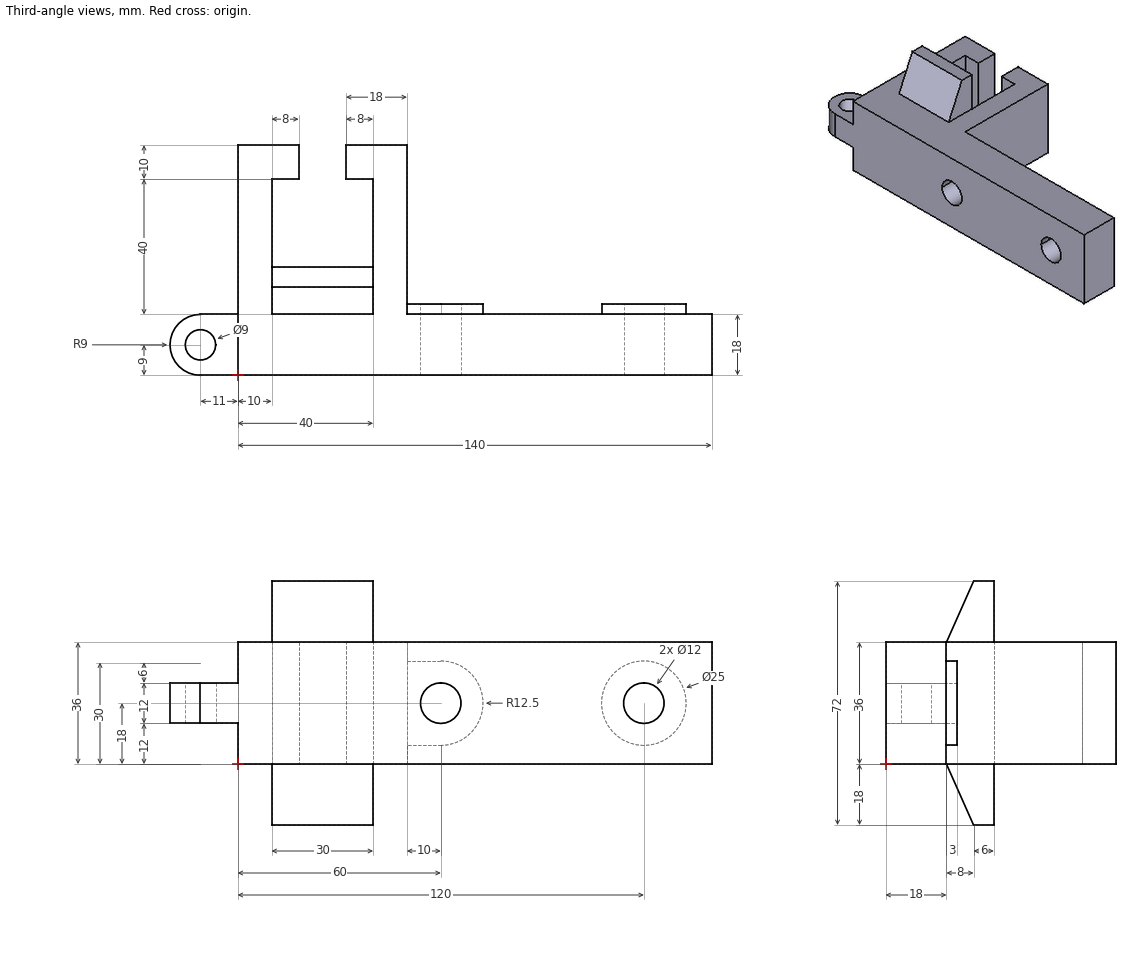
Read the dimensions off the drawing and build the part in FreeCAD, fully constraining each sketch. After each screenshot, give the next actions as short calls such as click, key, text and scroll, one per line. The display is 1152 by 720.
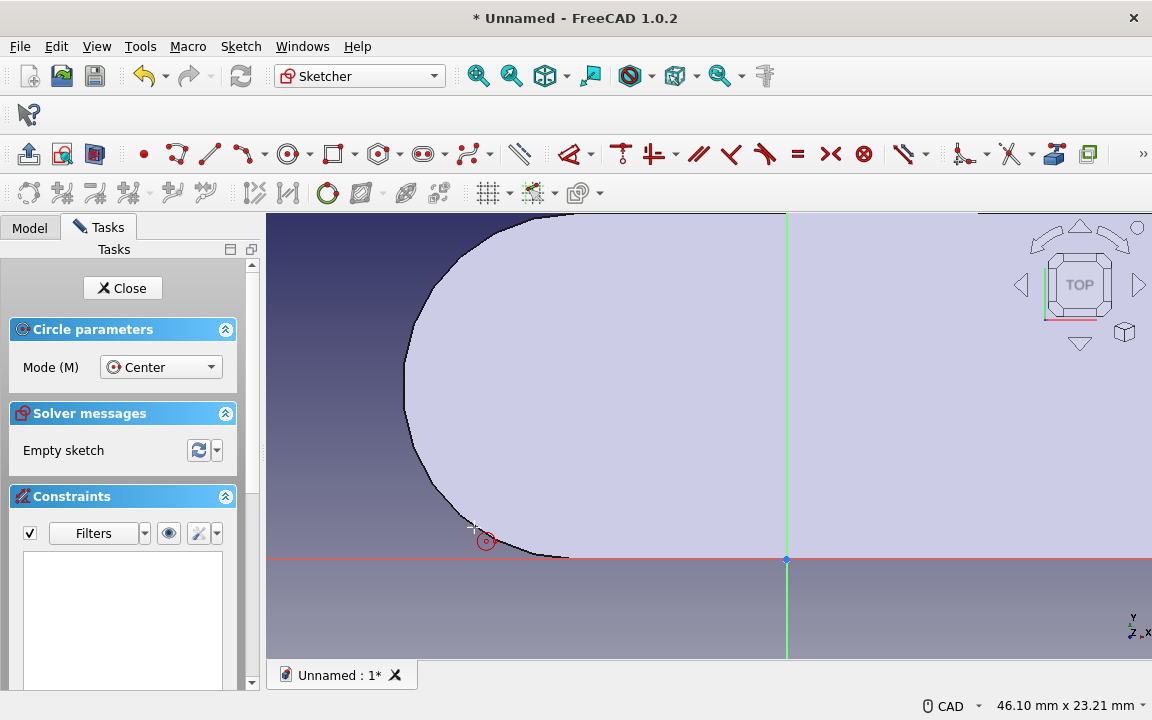
click(575, 386)
click(636, 325)
key(Escape)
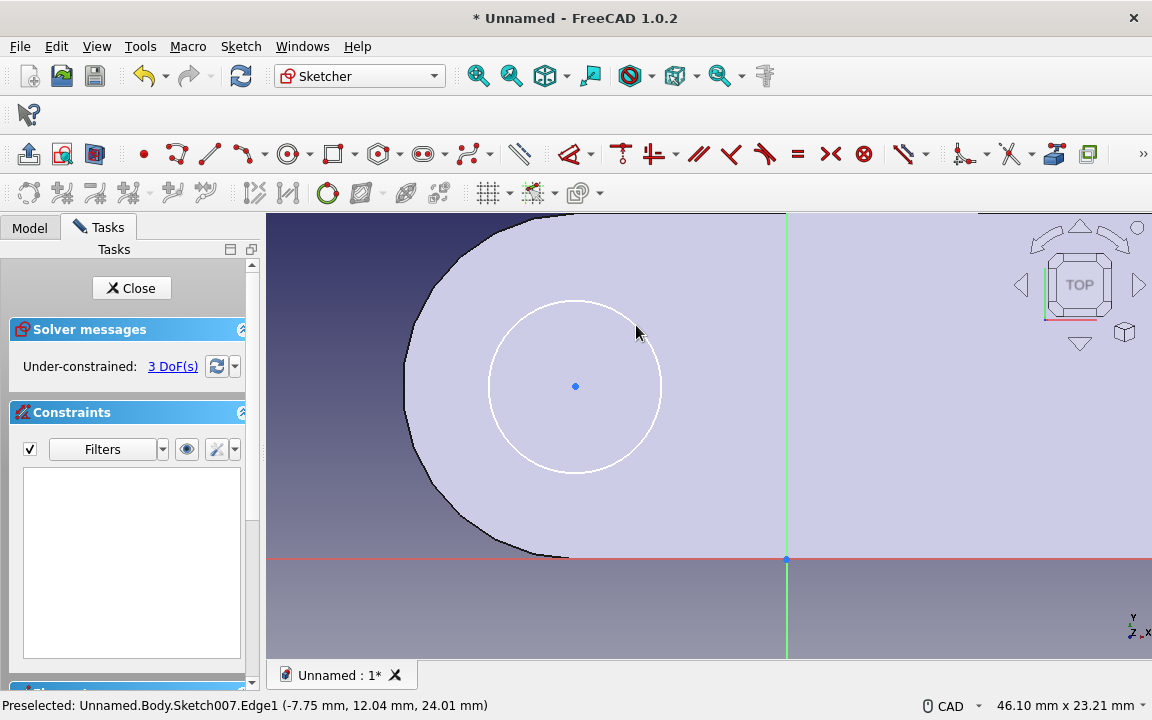
click(568, 154)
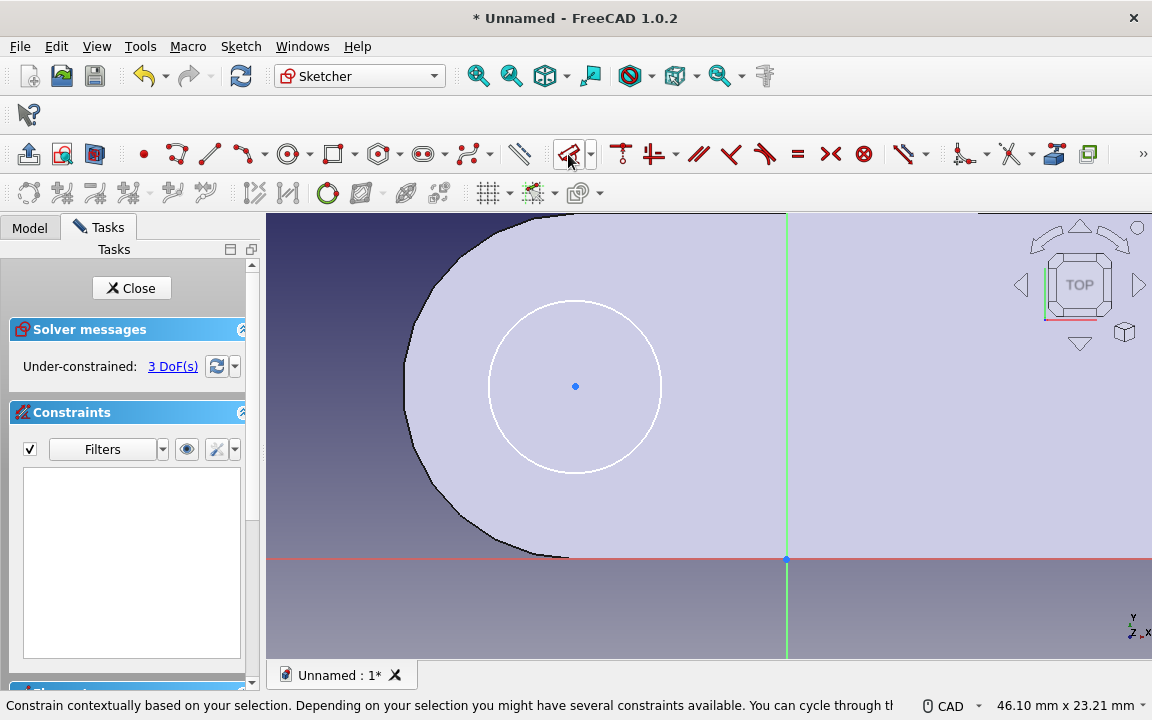
click(636, 326)
click(659, 303)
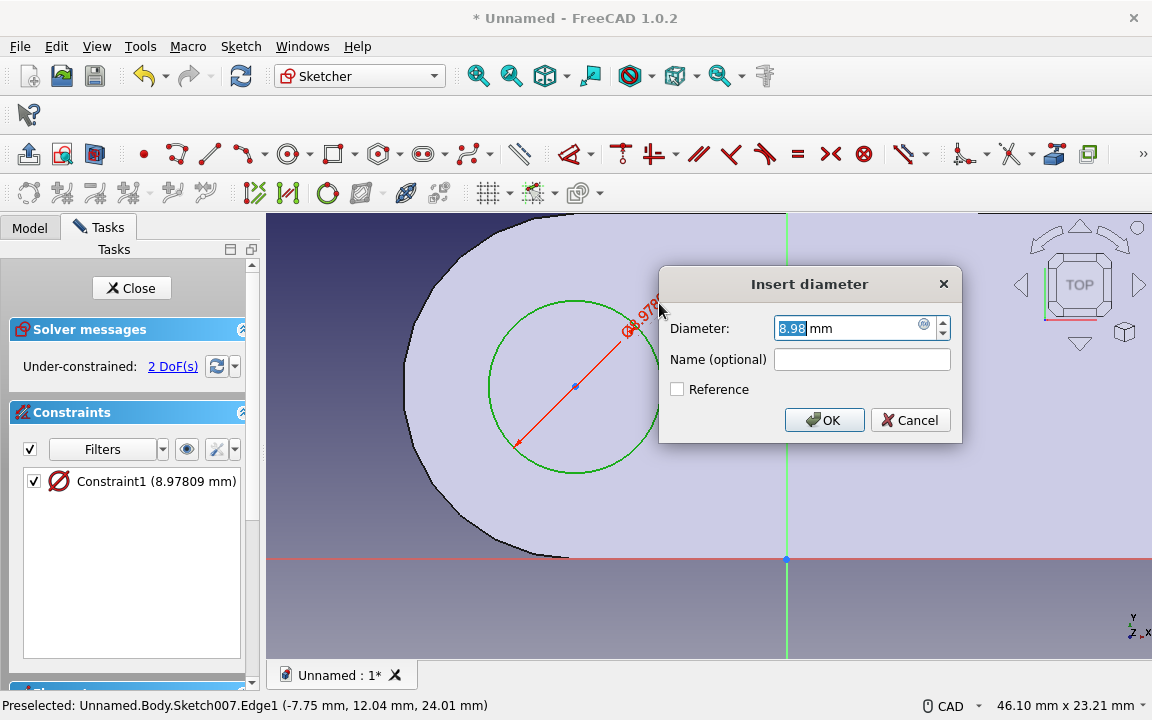
text(9)
key(Return)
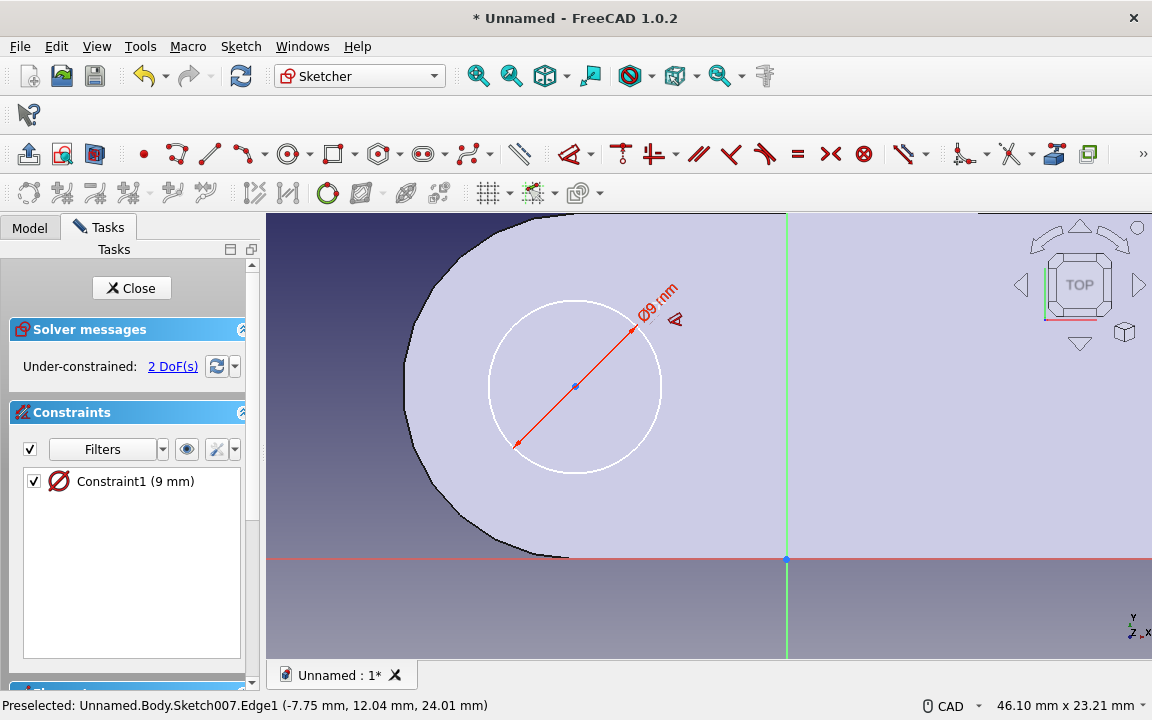
click(575, 387)
click(821, 473)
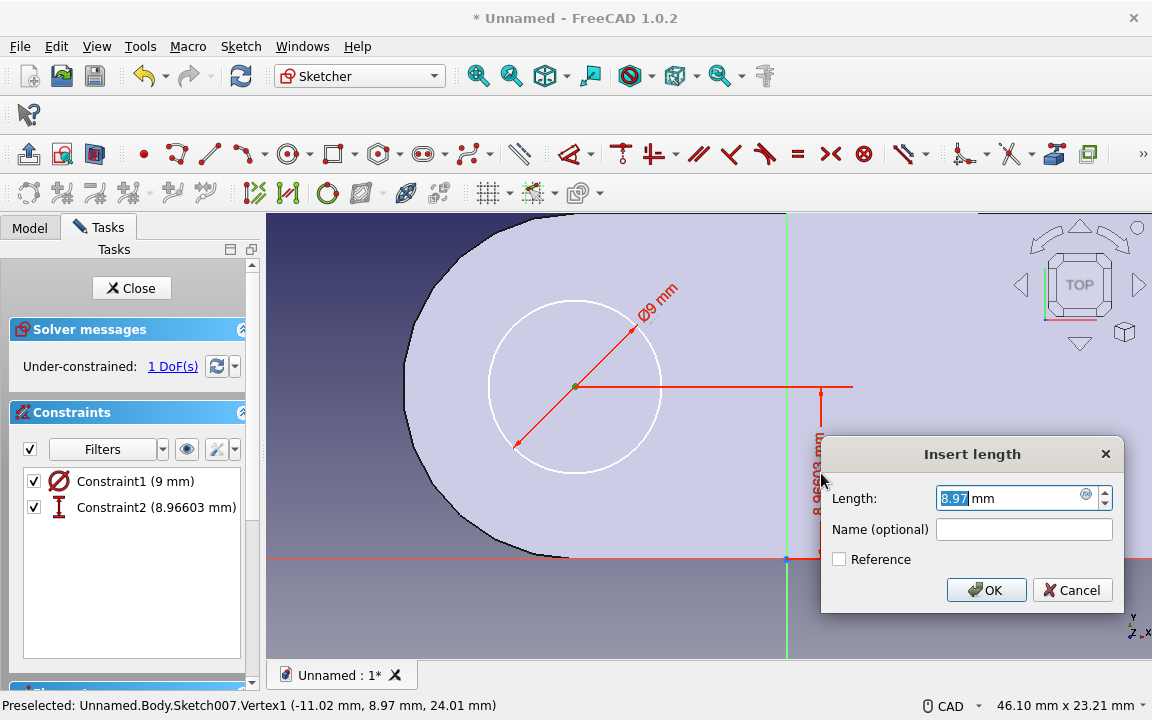
text(9)
key(Return)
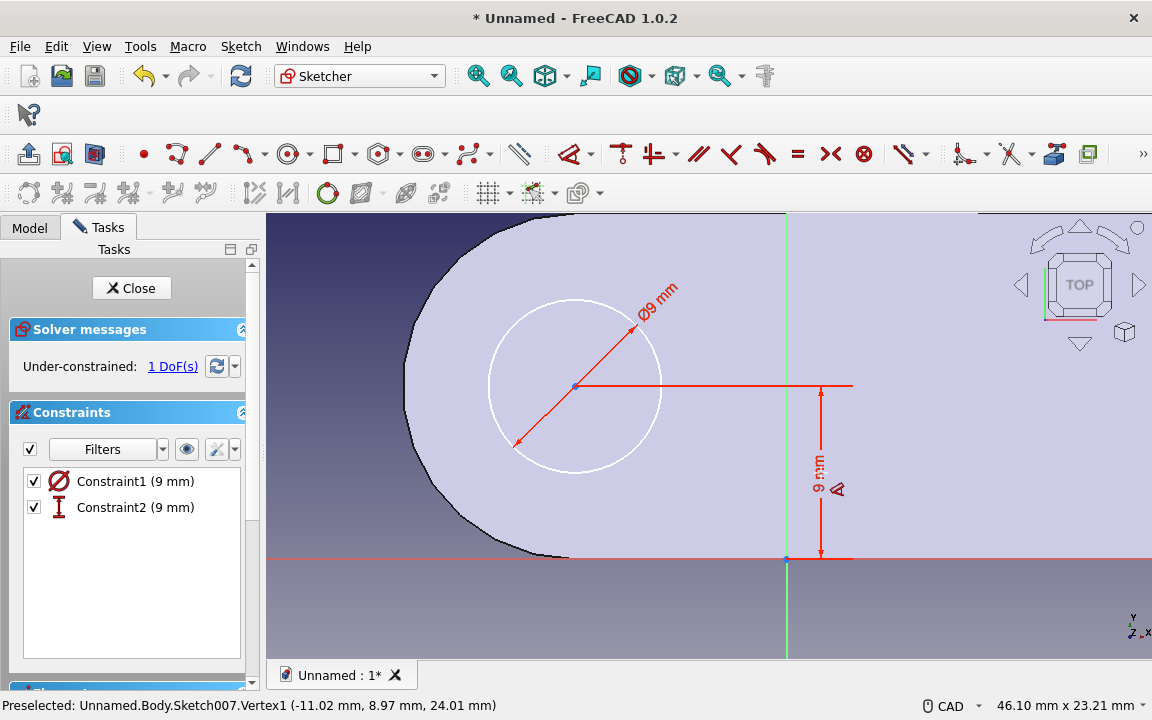
click(575, 386)
click(681, 593)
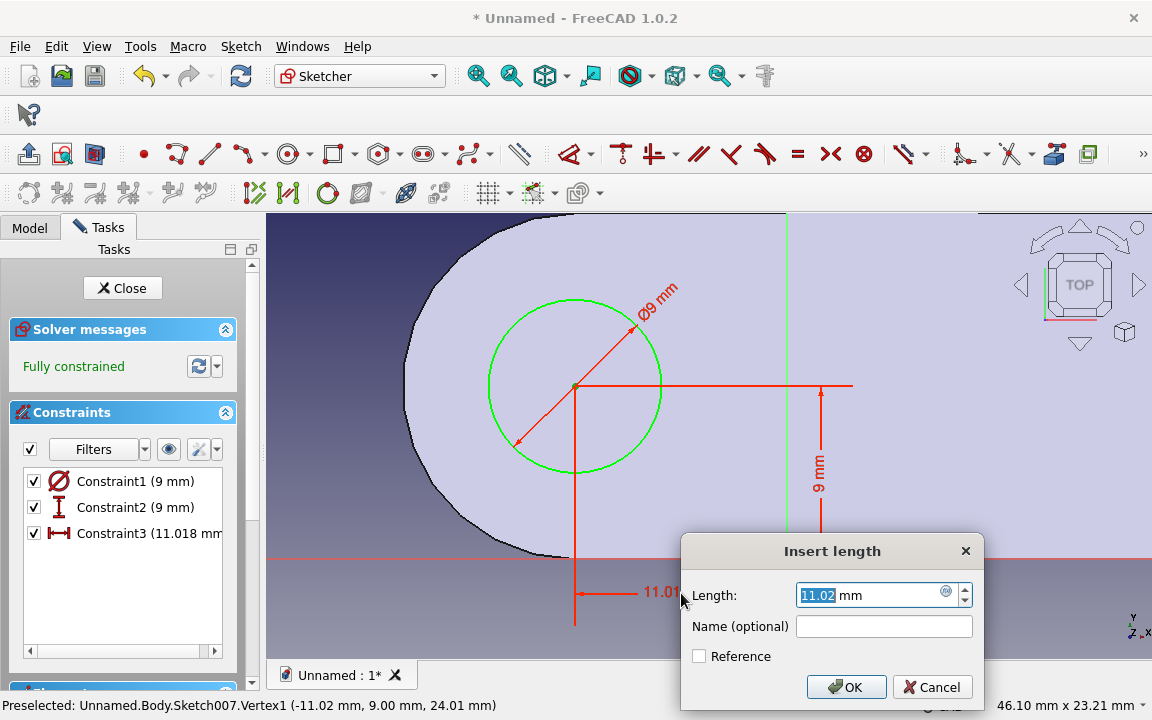
text(11)
key(Return)
key(Escape)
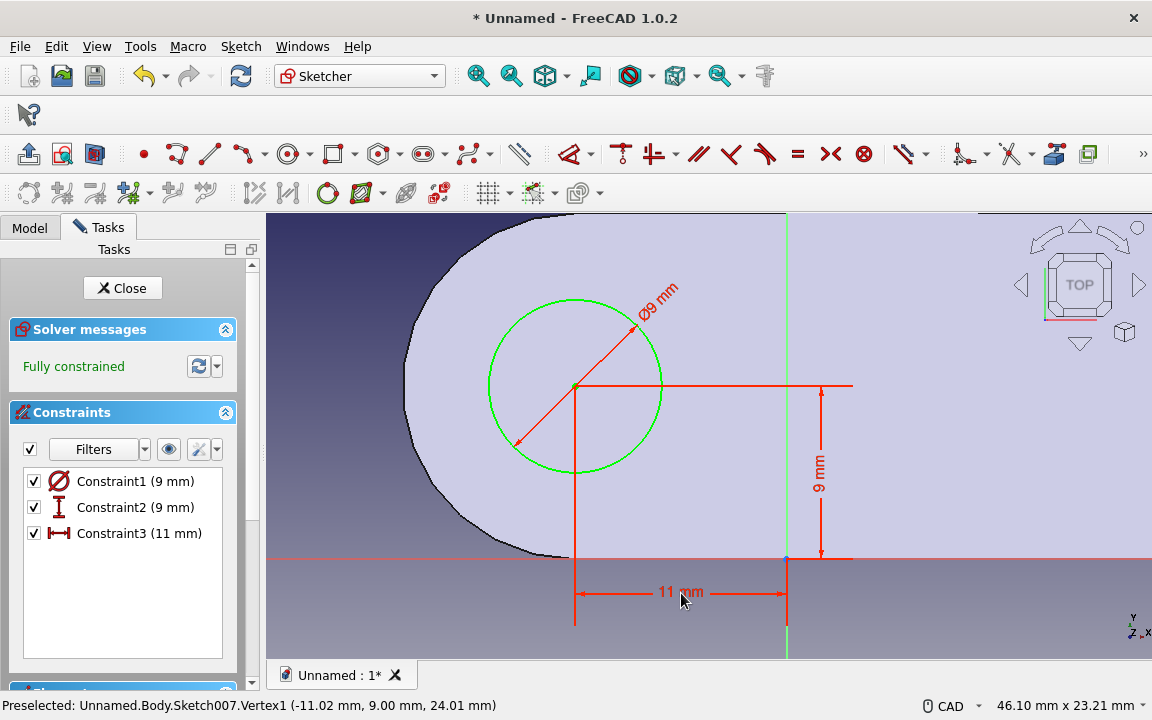
click(123, 288)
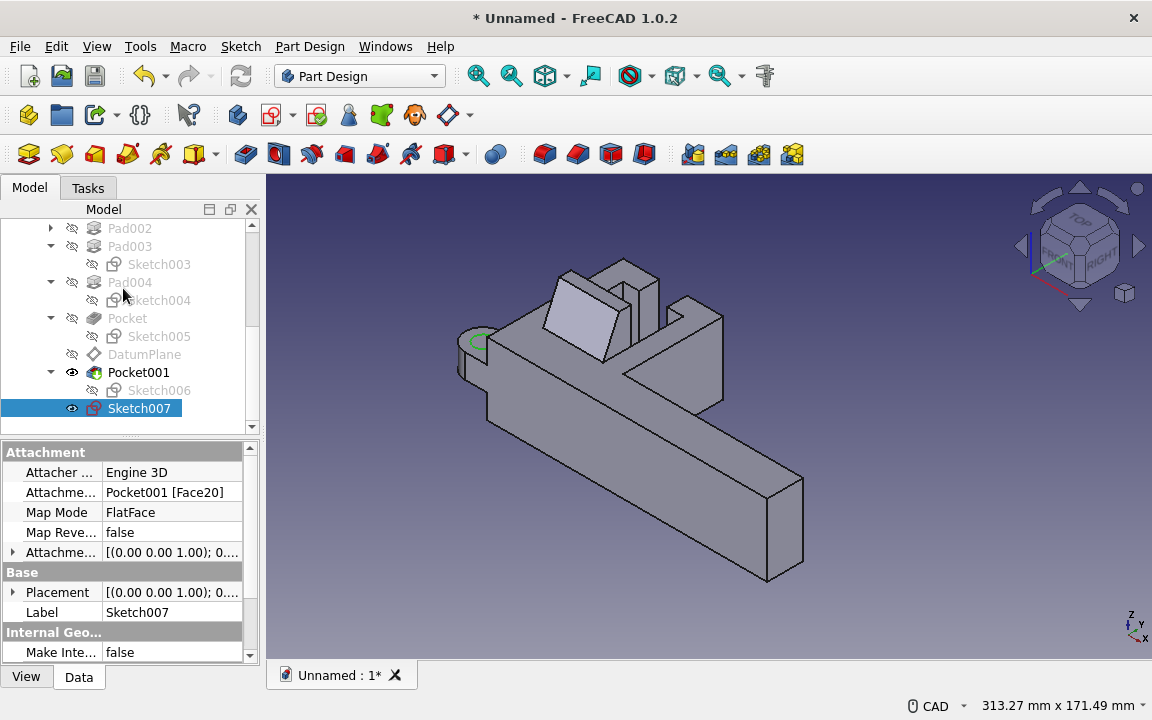
click(246, 154)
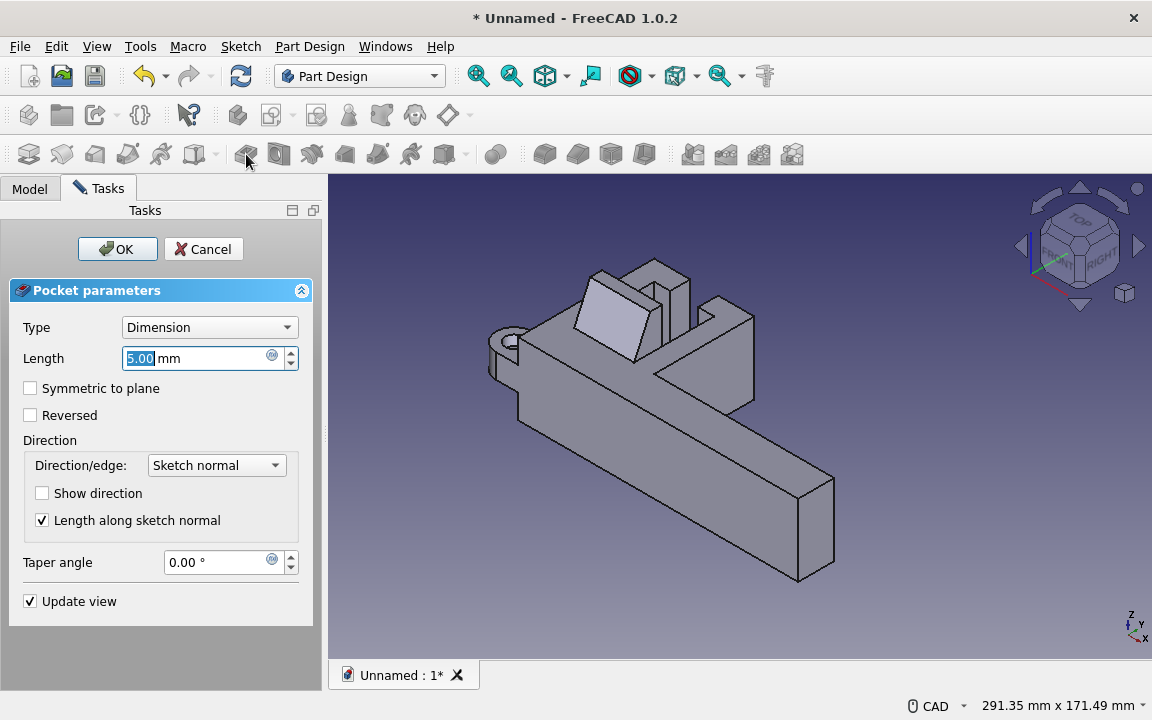
text(12)
key(Tab)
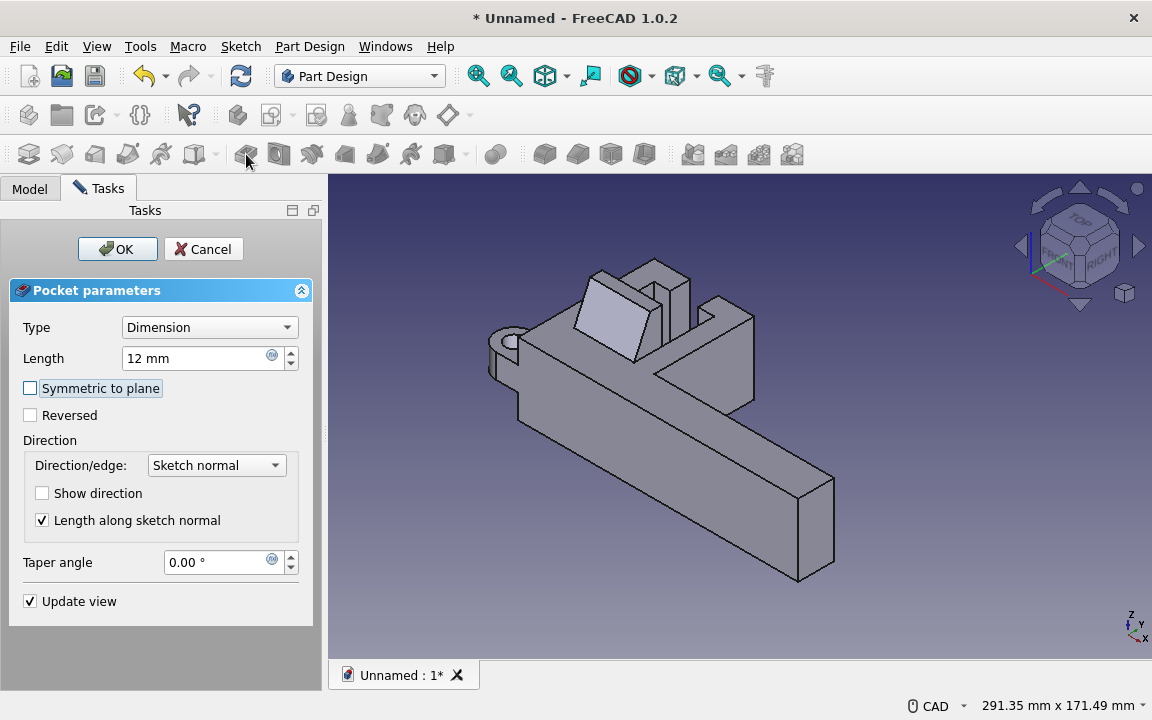
click(118, 249)